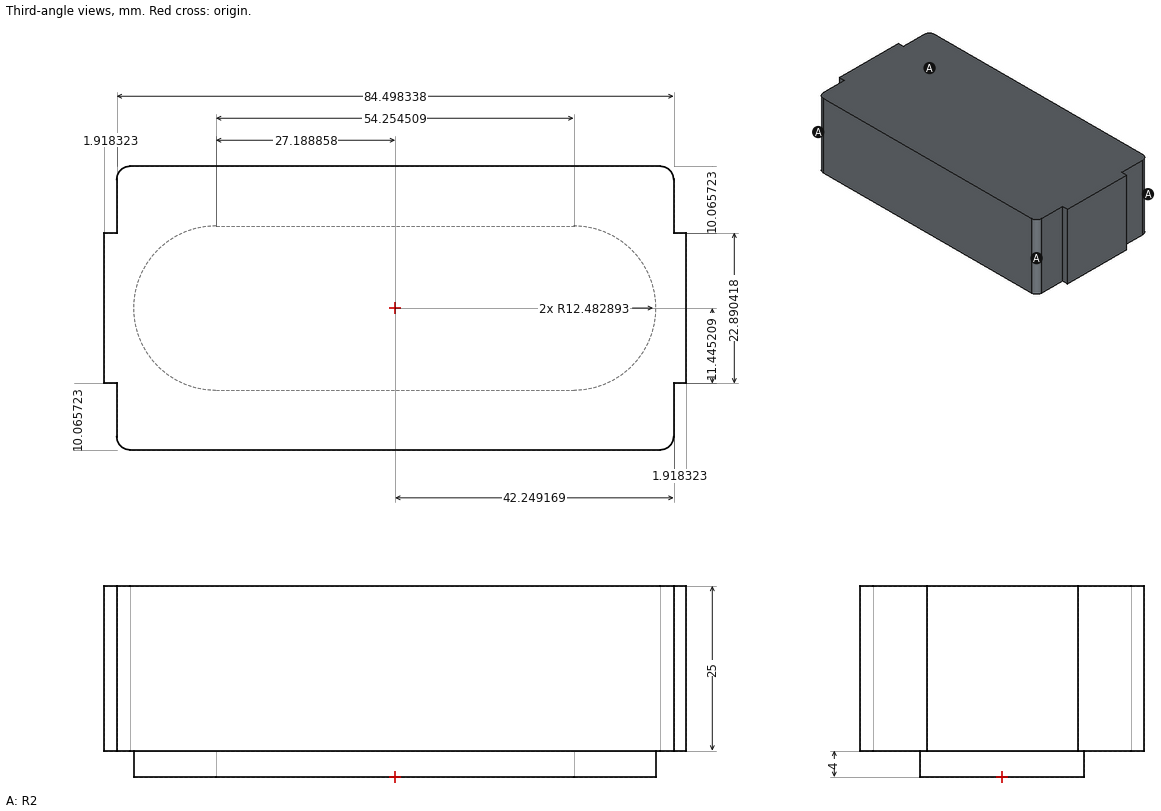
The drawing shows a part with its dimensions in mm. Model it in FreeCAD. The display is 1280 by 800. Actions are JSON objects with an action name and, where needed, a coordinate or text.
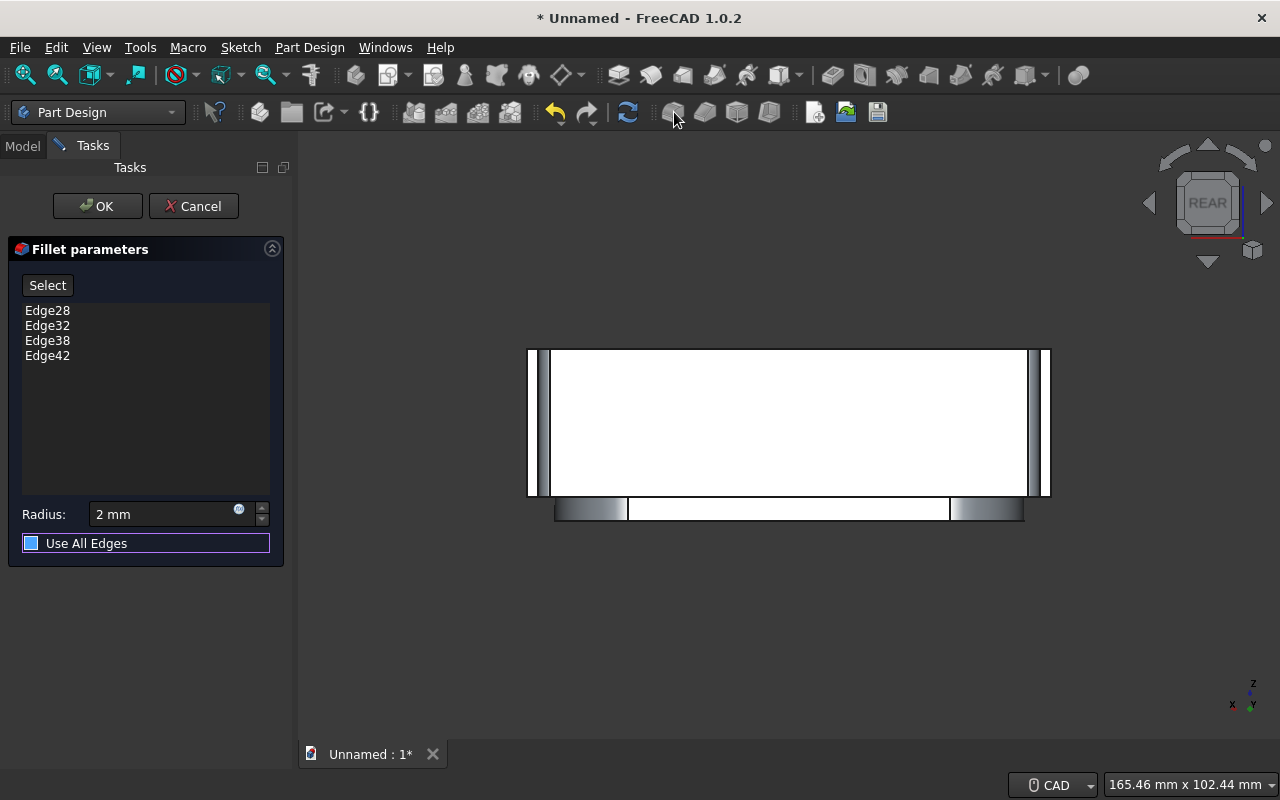
{"action": "left_click", "coordinate": [98, 206]}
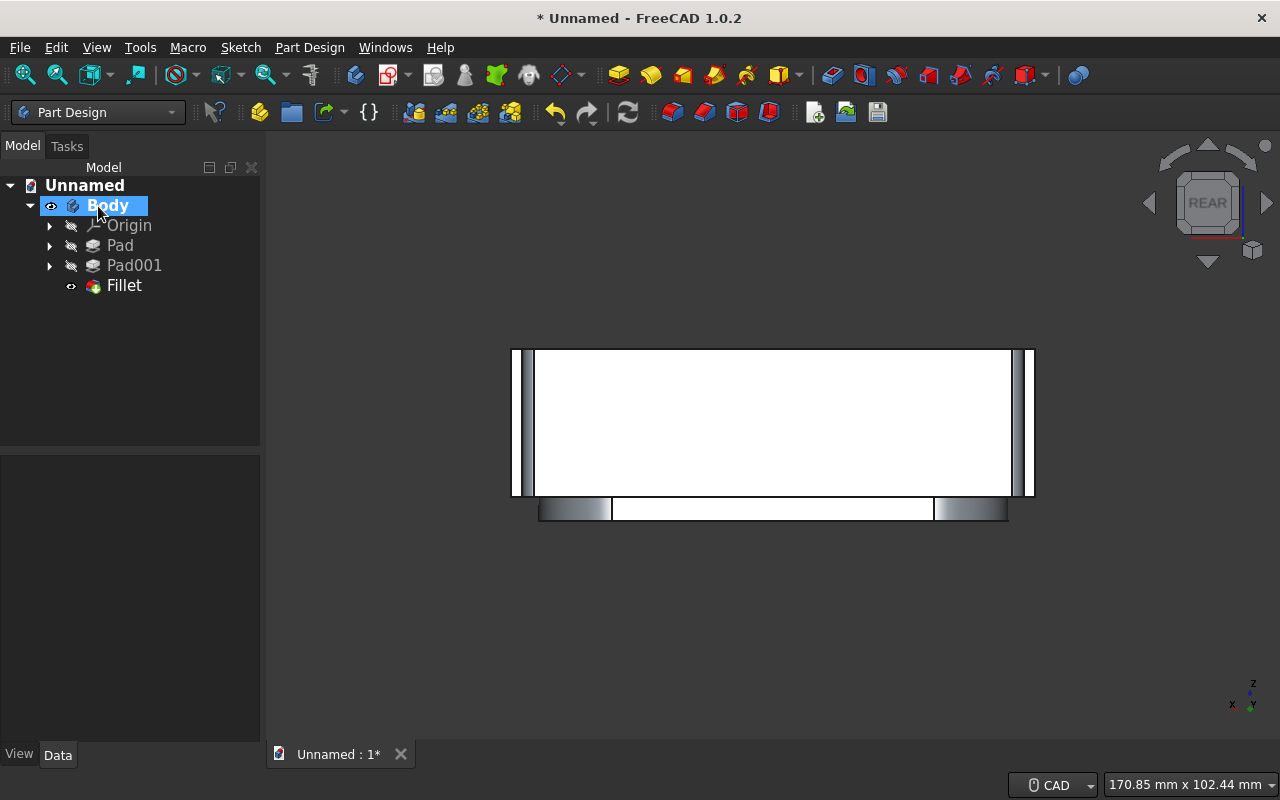
{"action": "key", "text": "0"}